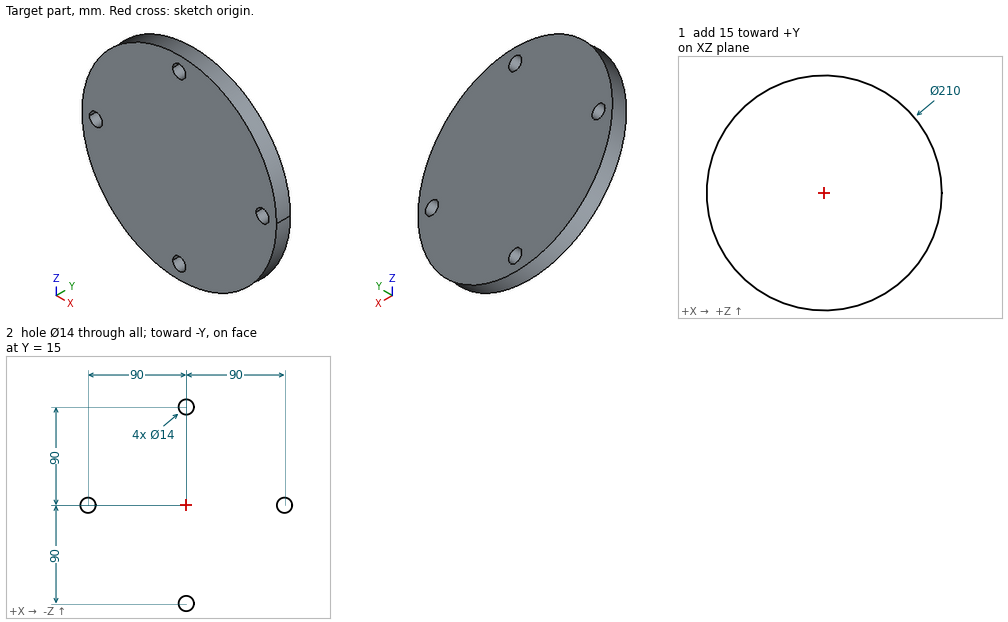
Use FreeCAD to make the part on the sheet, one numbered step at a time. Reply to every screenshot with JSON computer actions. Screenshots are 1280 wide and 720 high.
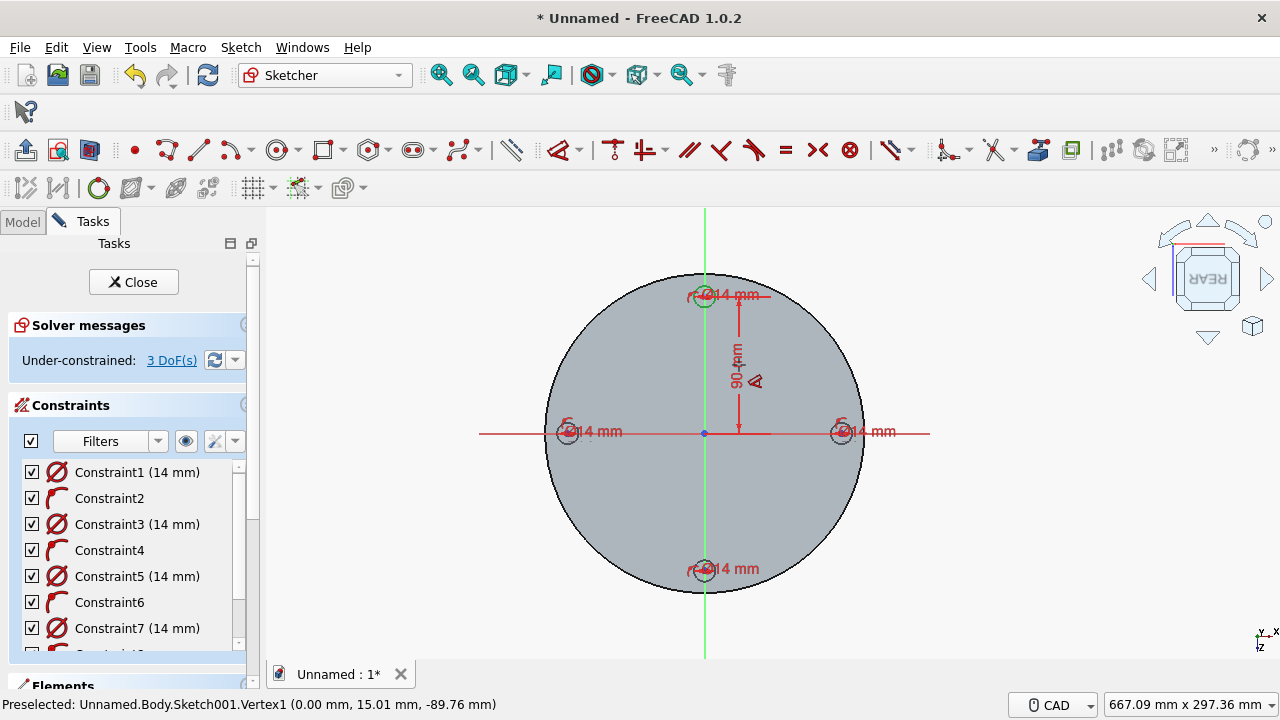
{"action": "left_click", "coordinate": [842, 434]}
{"action": "left_click", "coordinate": [773, 468]}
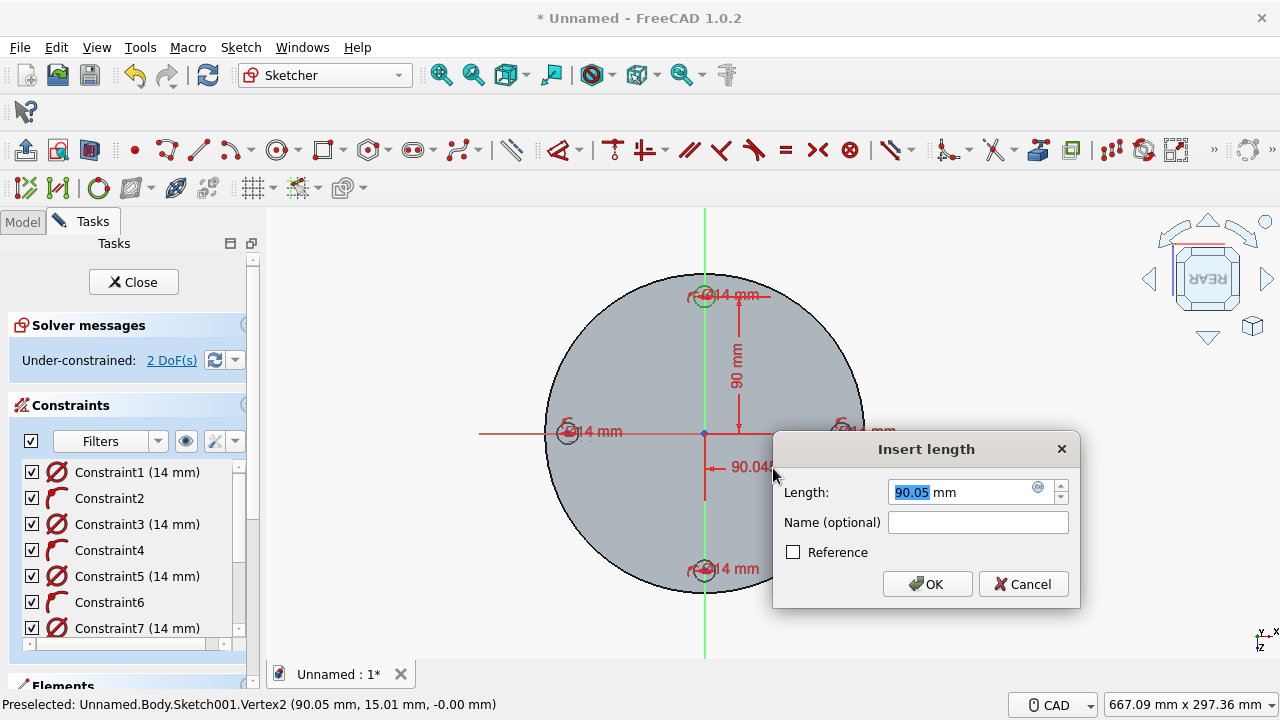
{"action": "type", "text": "90"}
{"action": "key", "text": "Return"}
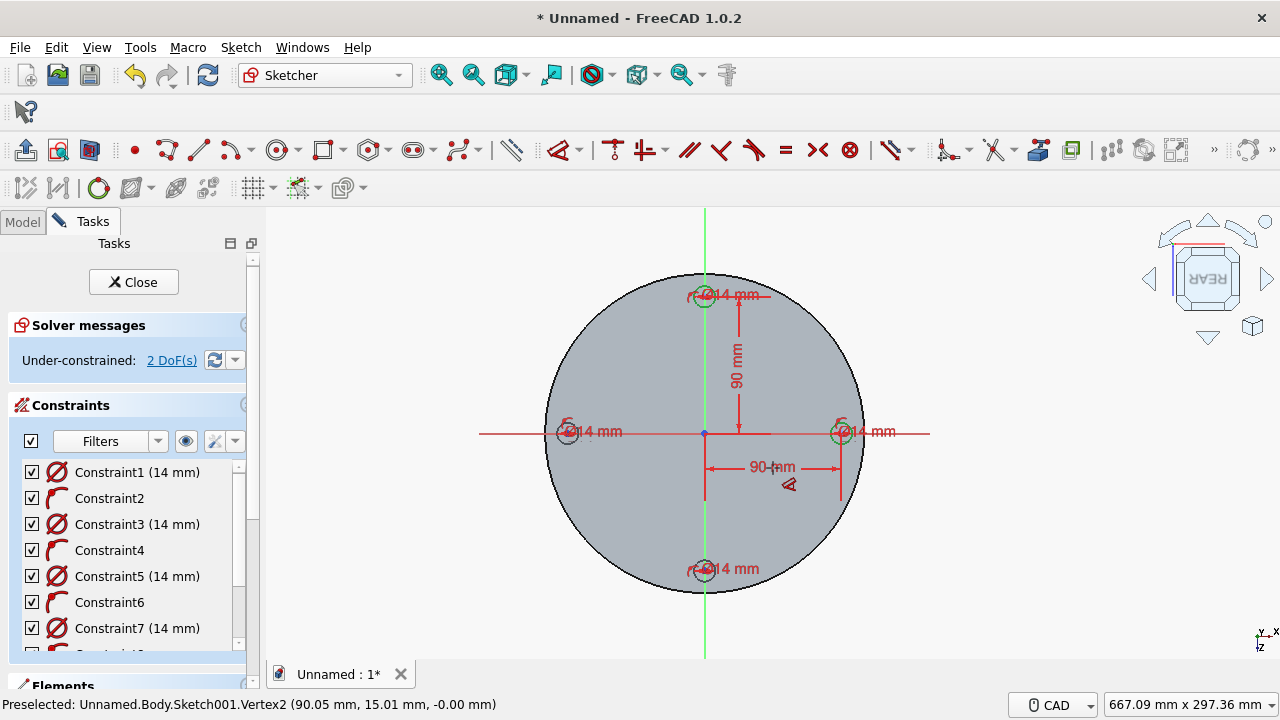
{"action": "left_click", "coordinate": [705, 571]}
{"action": "left_click", "coordinate": [739, 502]}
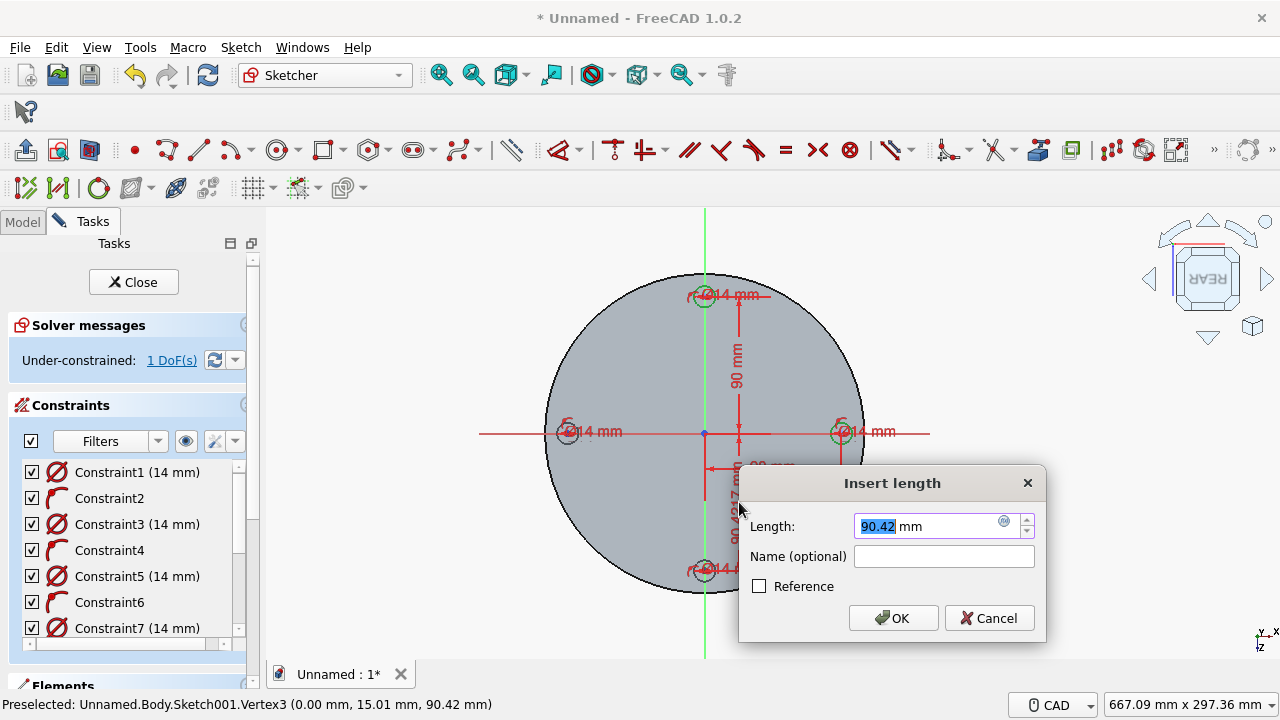
{"action": "type", "text": "90"}
{"action": "key", "text": "Return"}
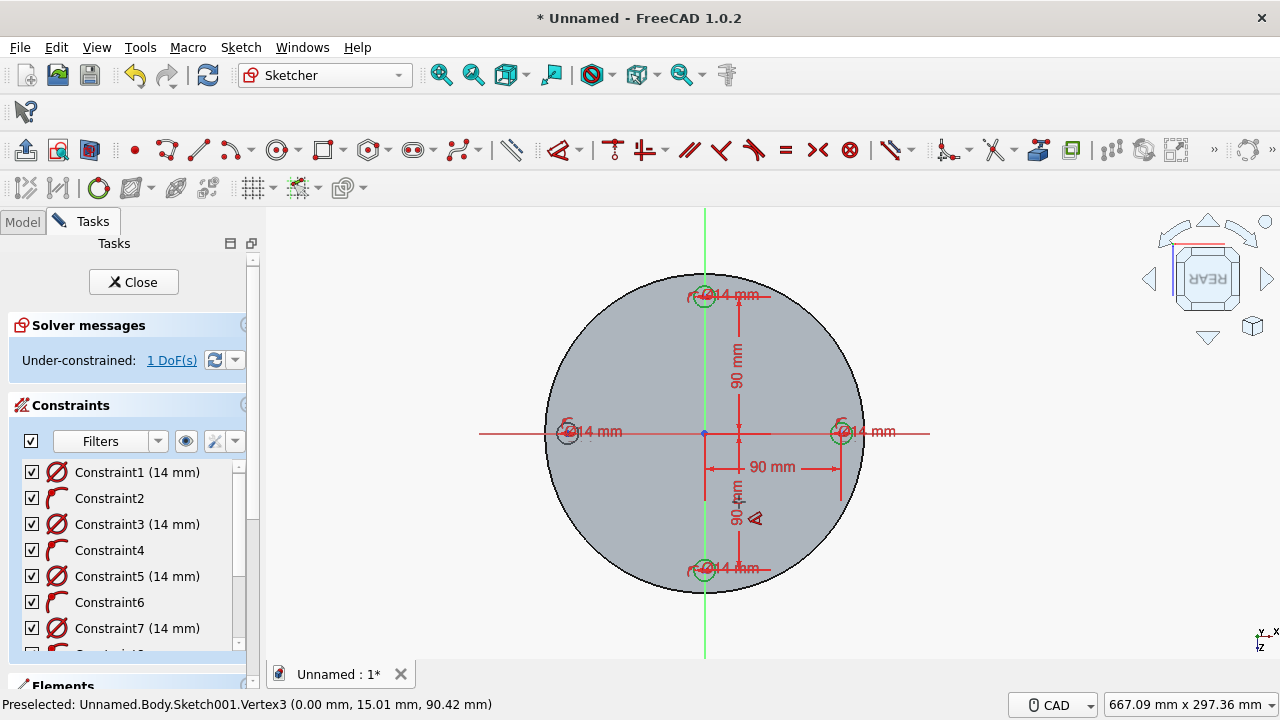
{"action": "left_click", "coordinate": [568, 434]}
{"action": "left_click", "coordinate": [636, 468]}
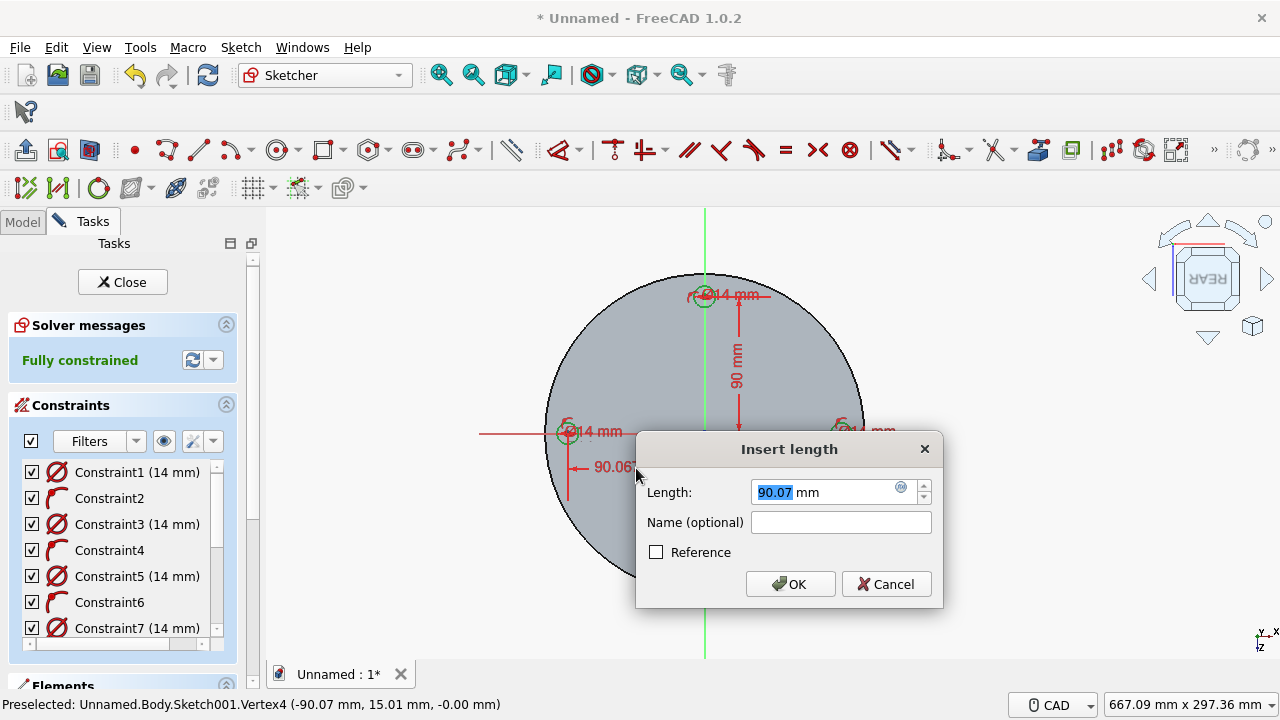
{"action": "type", "text": "90"}
{"action": "key", "text": "Return"}
{"action": "key", "text": "Escape"}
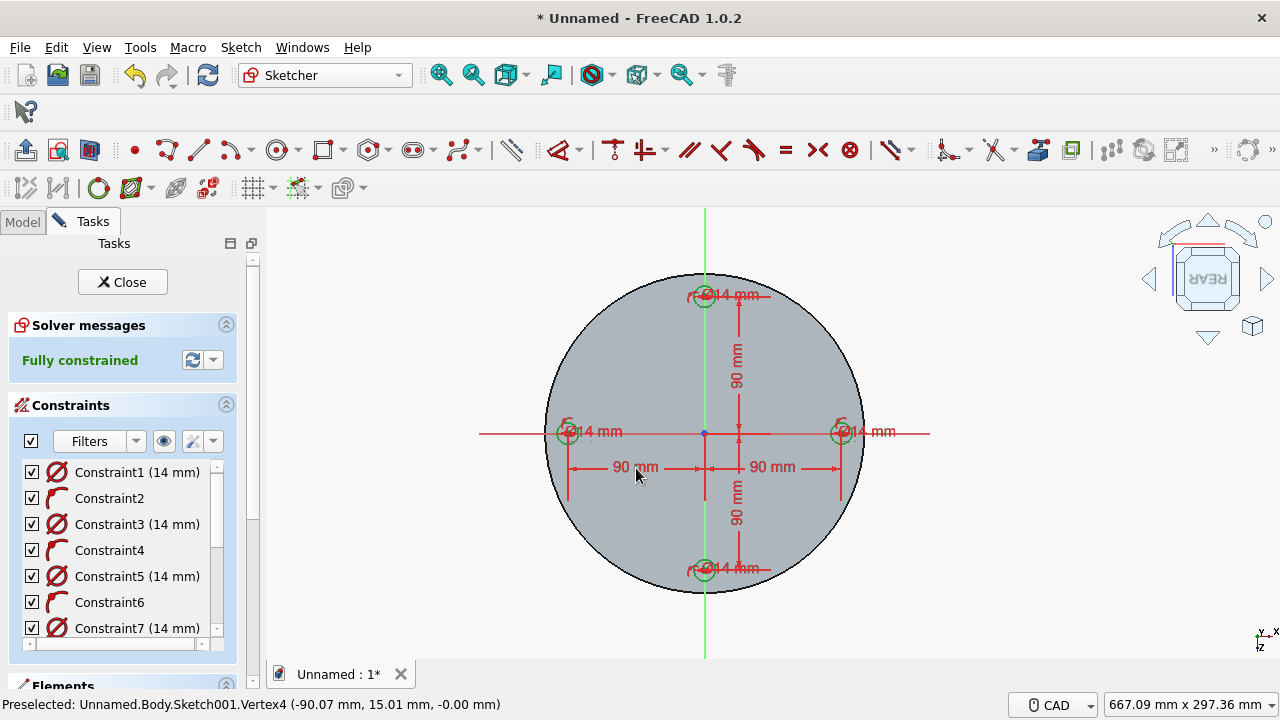
{"action": "left_click", "coordinate": [123, 282]}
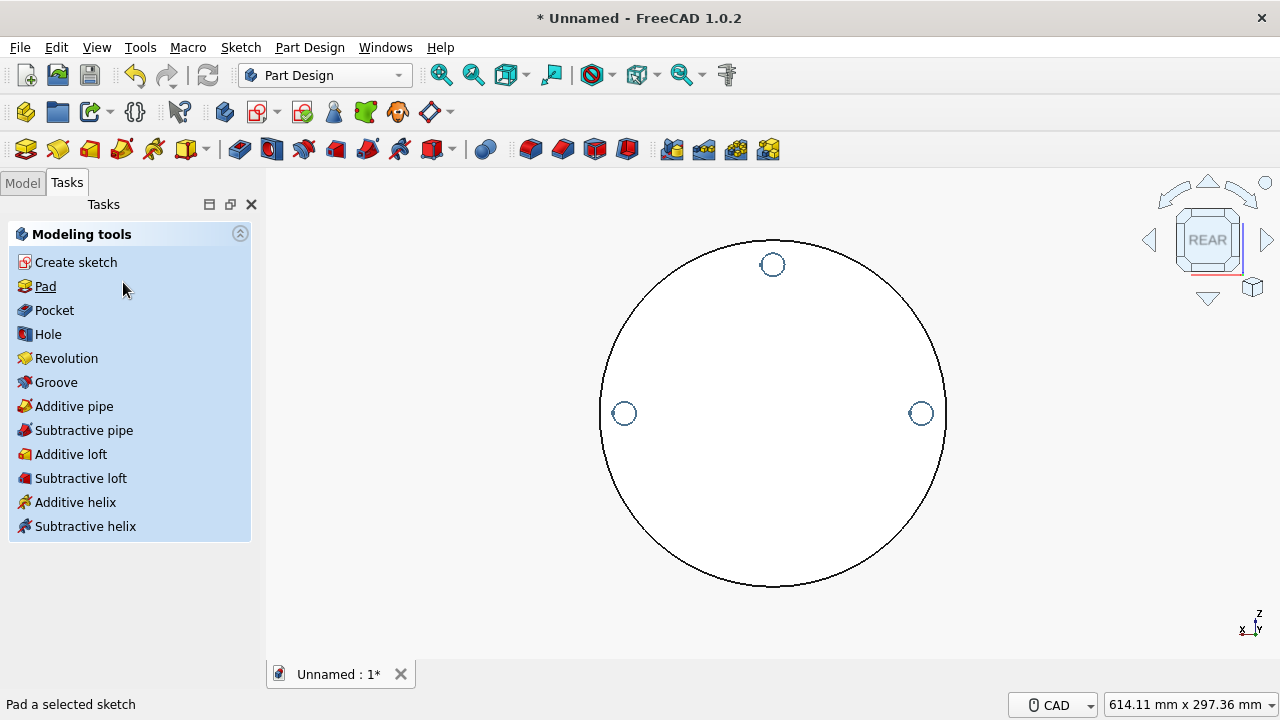
{"action": "left_click", "coordinate": [272, 150]}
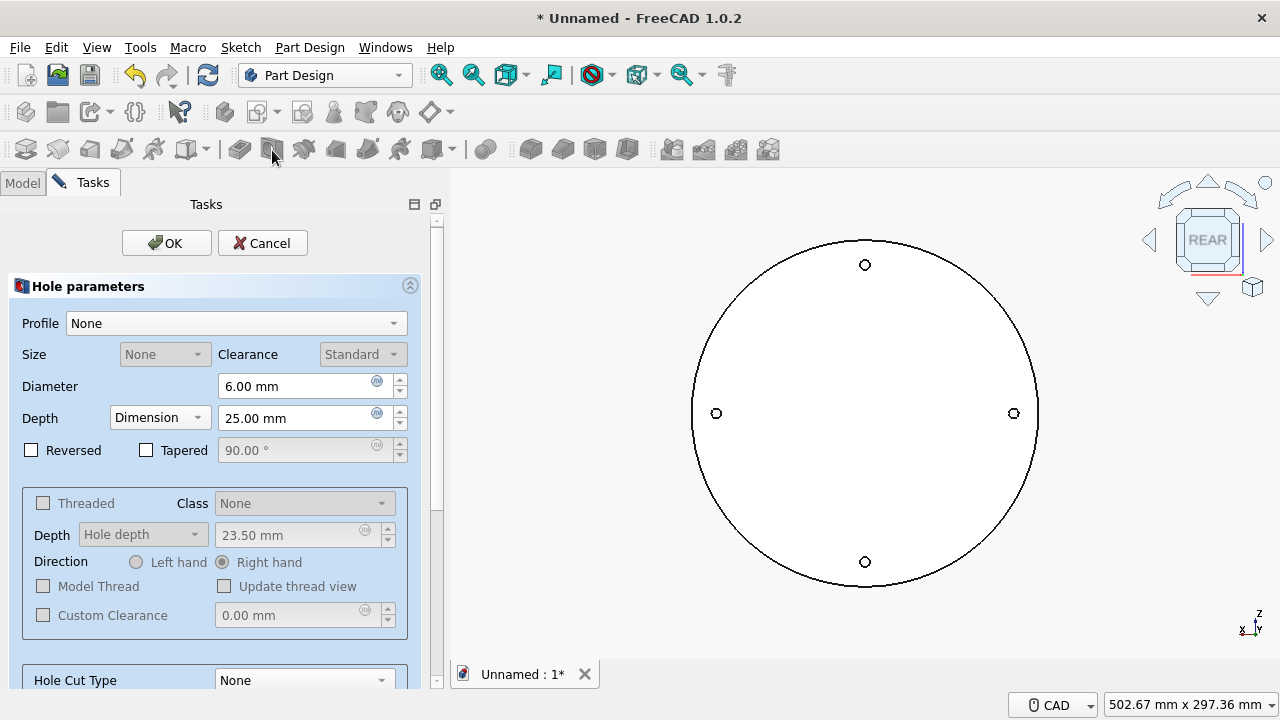
{"action": "triple_click", "coordinate": [305, 386]}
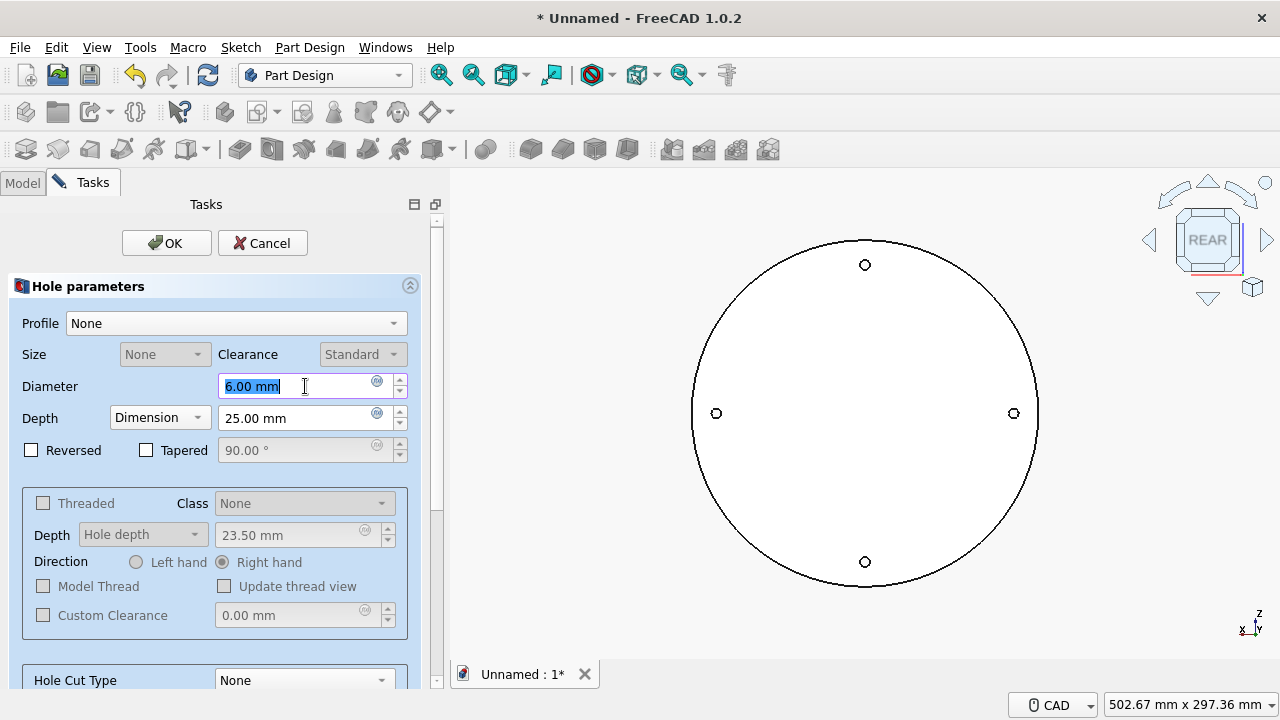
{"action": "type", "text": "14"}
{"action": "key", "text": "Tab"}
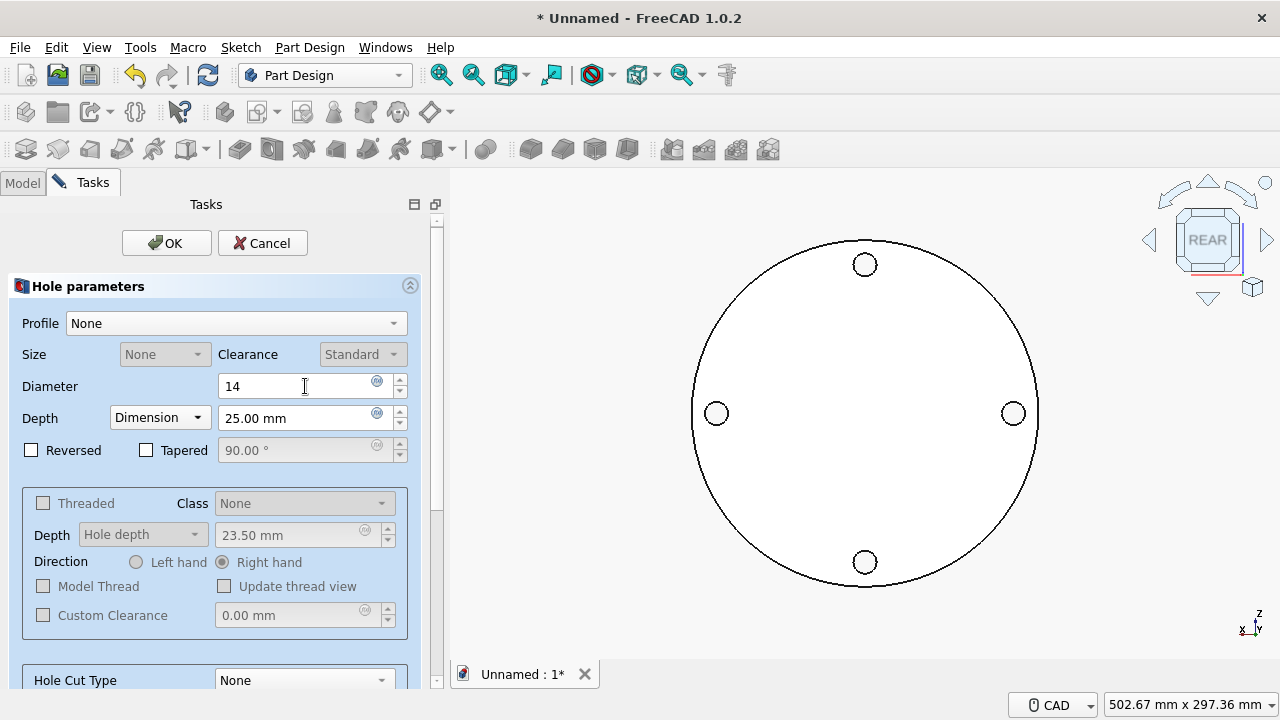
{"action": "left_click", "coordinate": [161, 418]}